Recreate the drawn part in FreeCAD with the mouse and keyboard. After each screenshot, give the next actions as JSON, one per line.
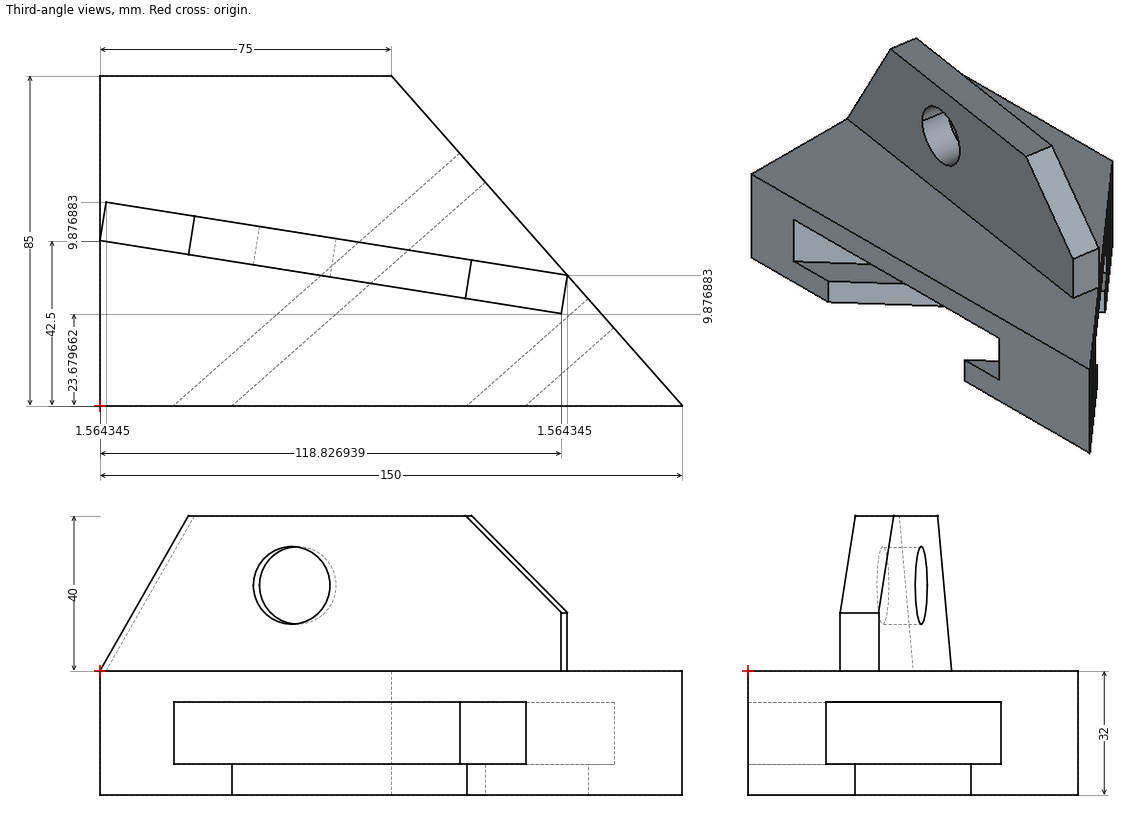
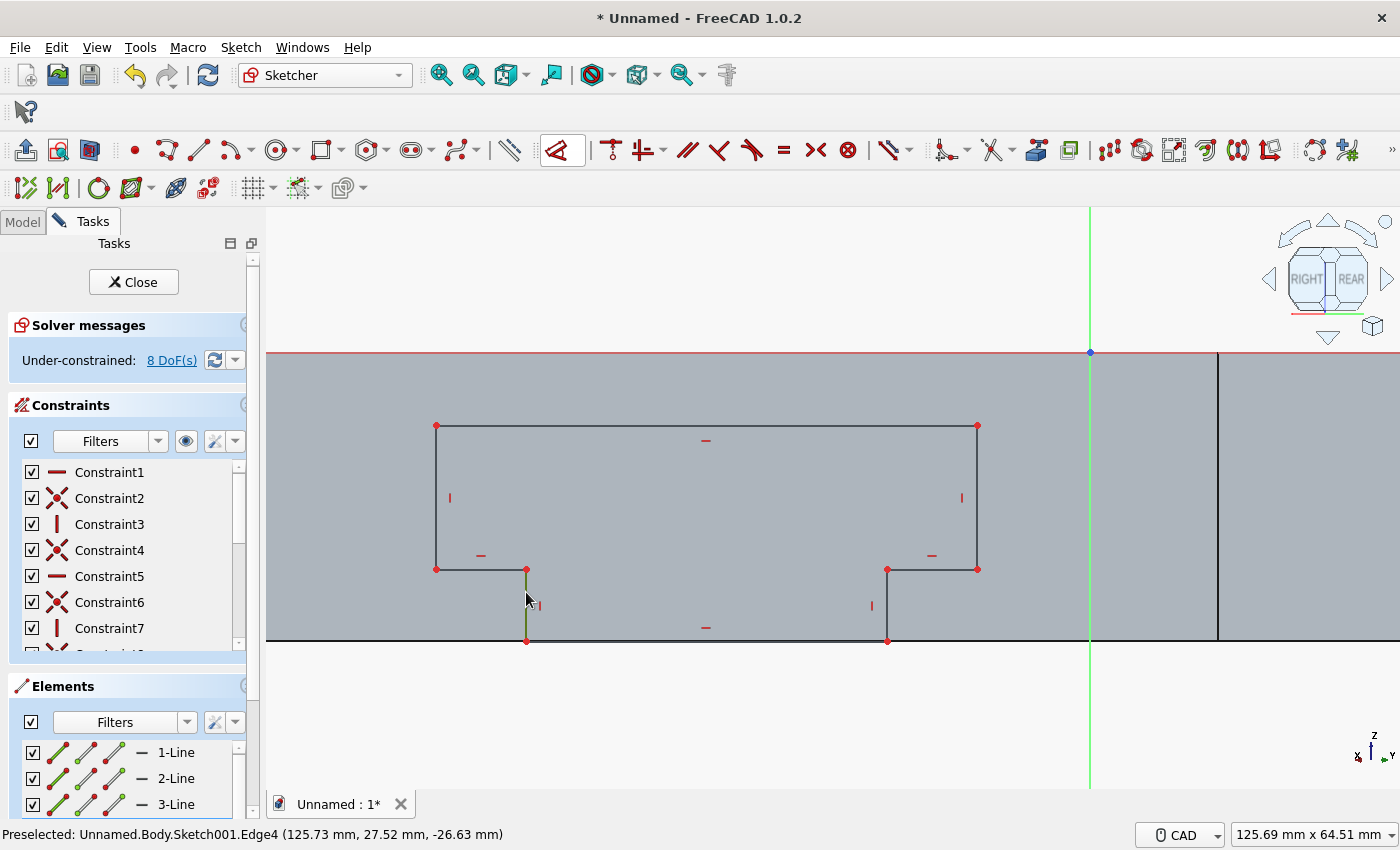
{"action": "key", "text": "i"}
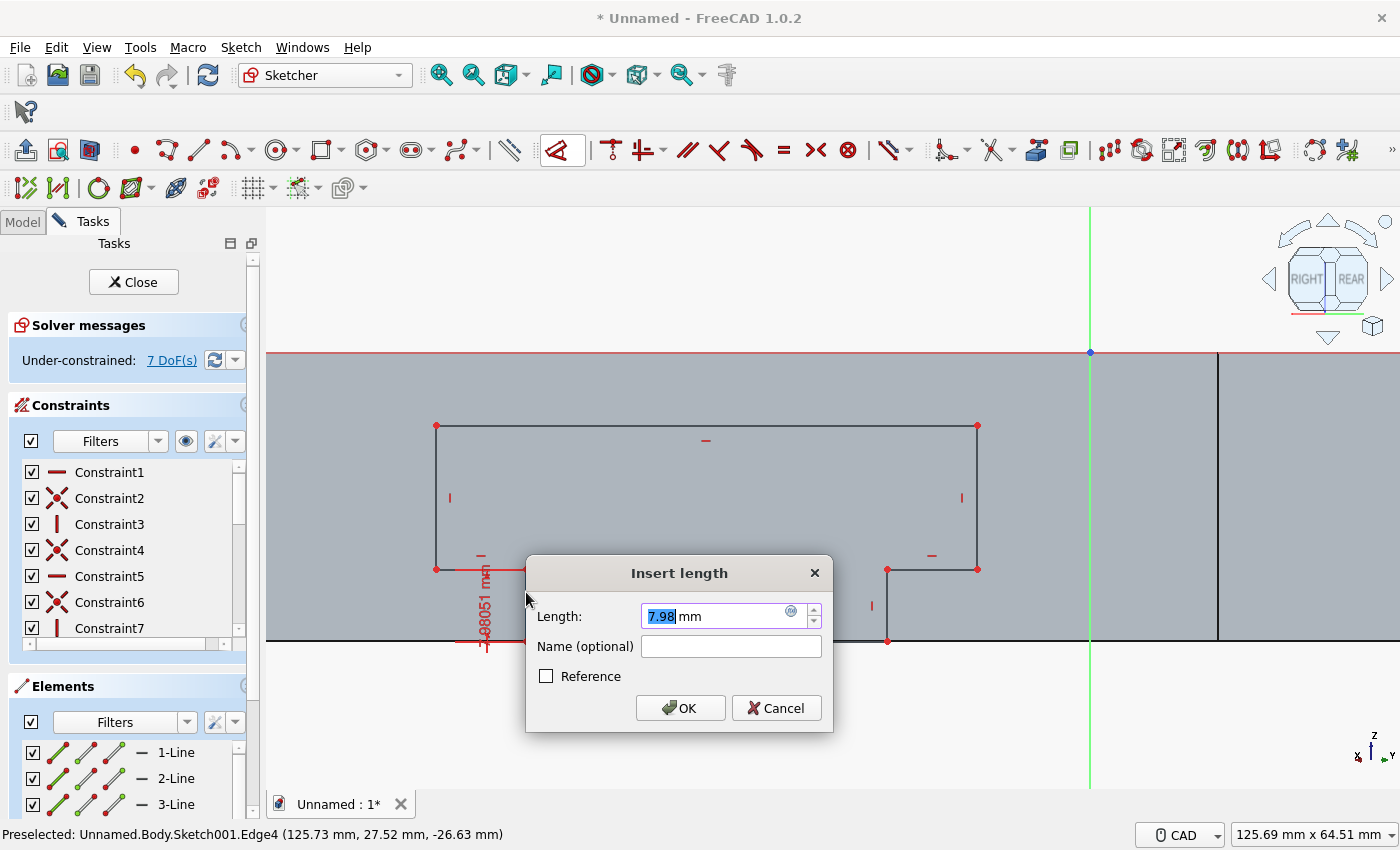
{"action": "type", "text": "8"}
{"action": "key", "text": "Return"}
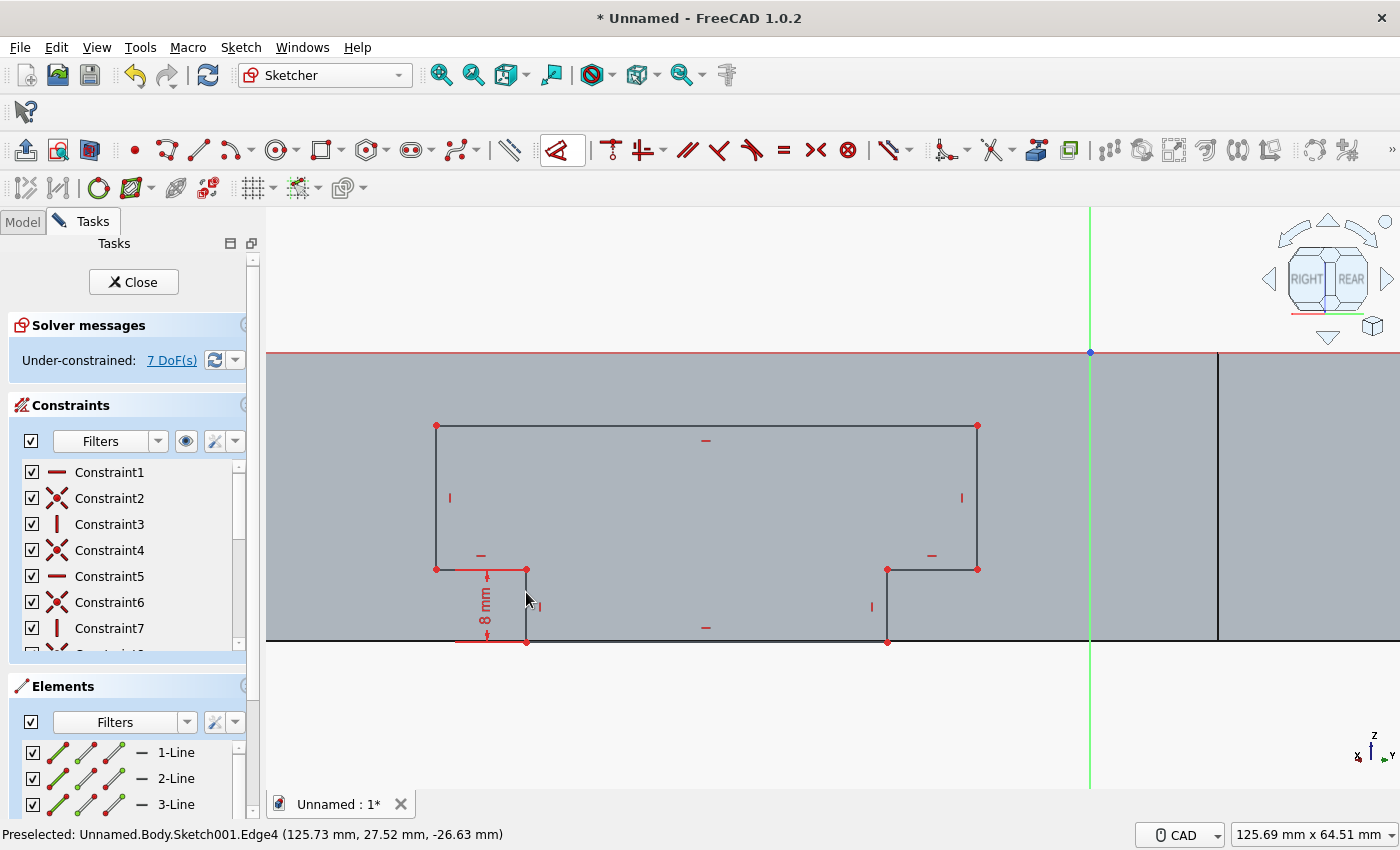
{"action": "left_click", "coordinate": [887, 621]}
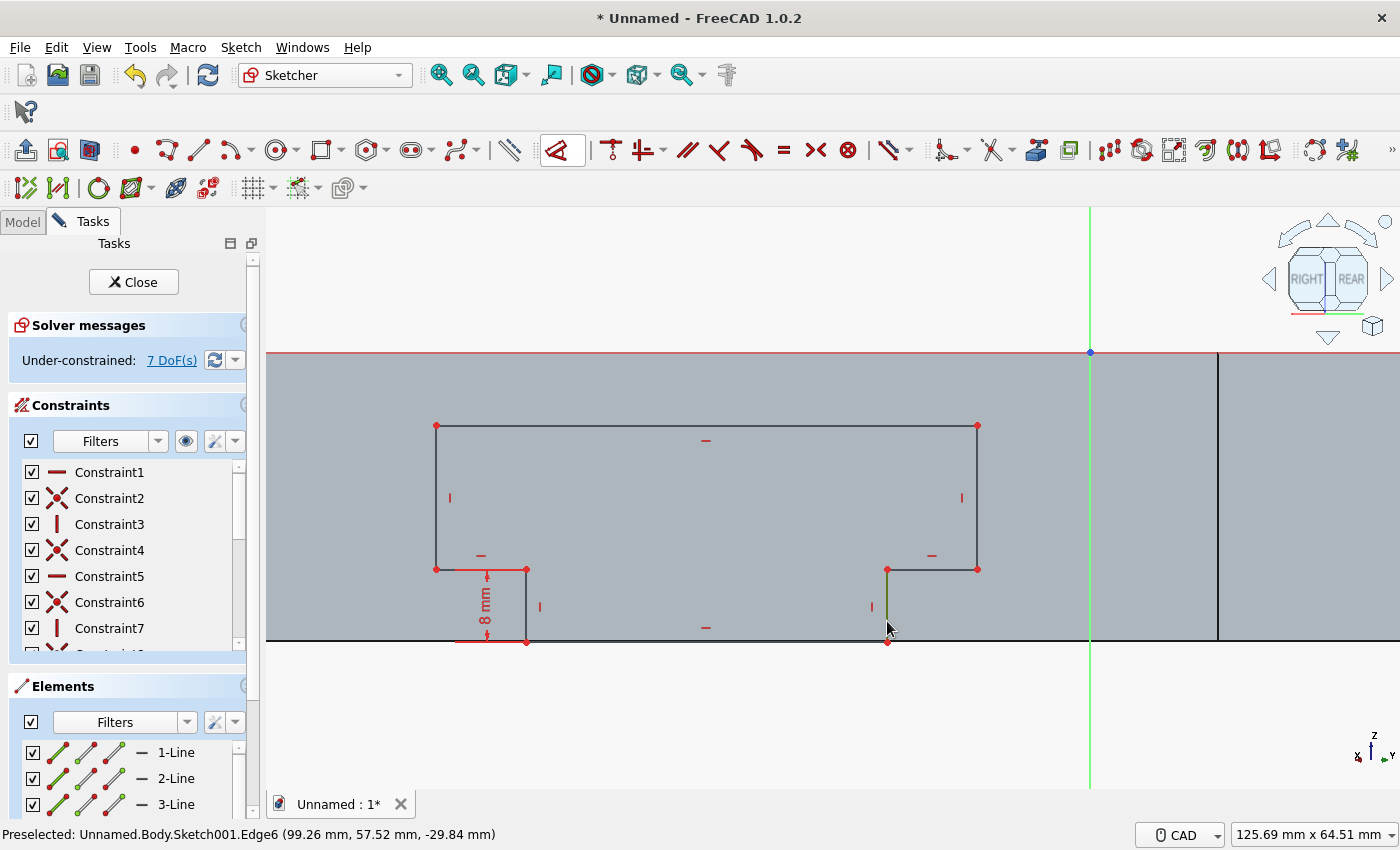
{"action": "key", "text": "i"}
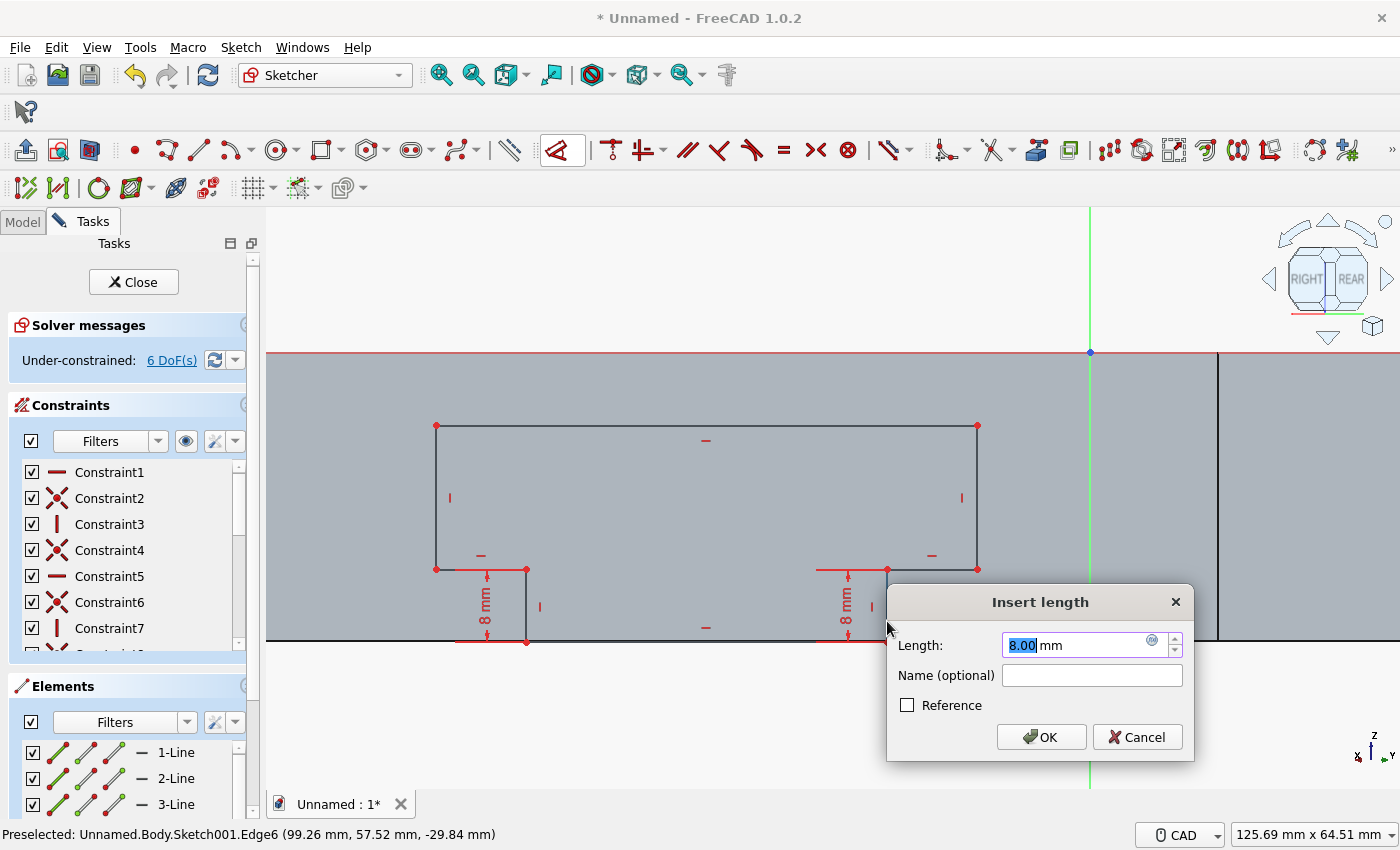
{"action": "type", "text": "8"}
{"action": "key", "text": "Return"}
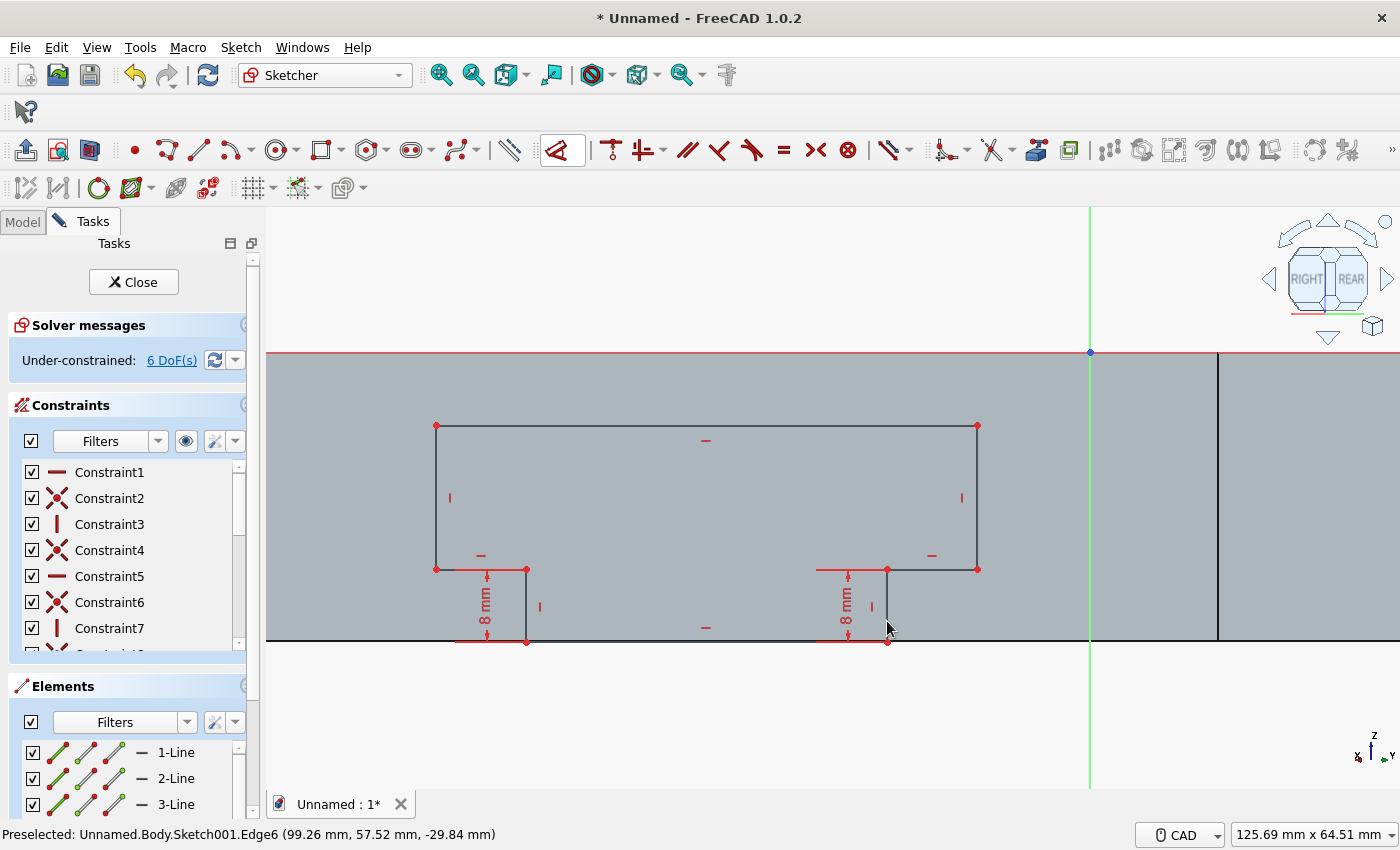
{"action": "left_click", "coordinate": [815, 426]}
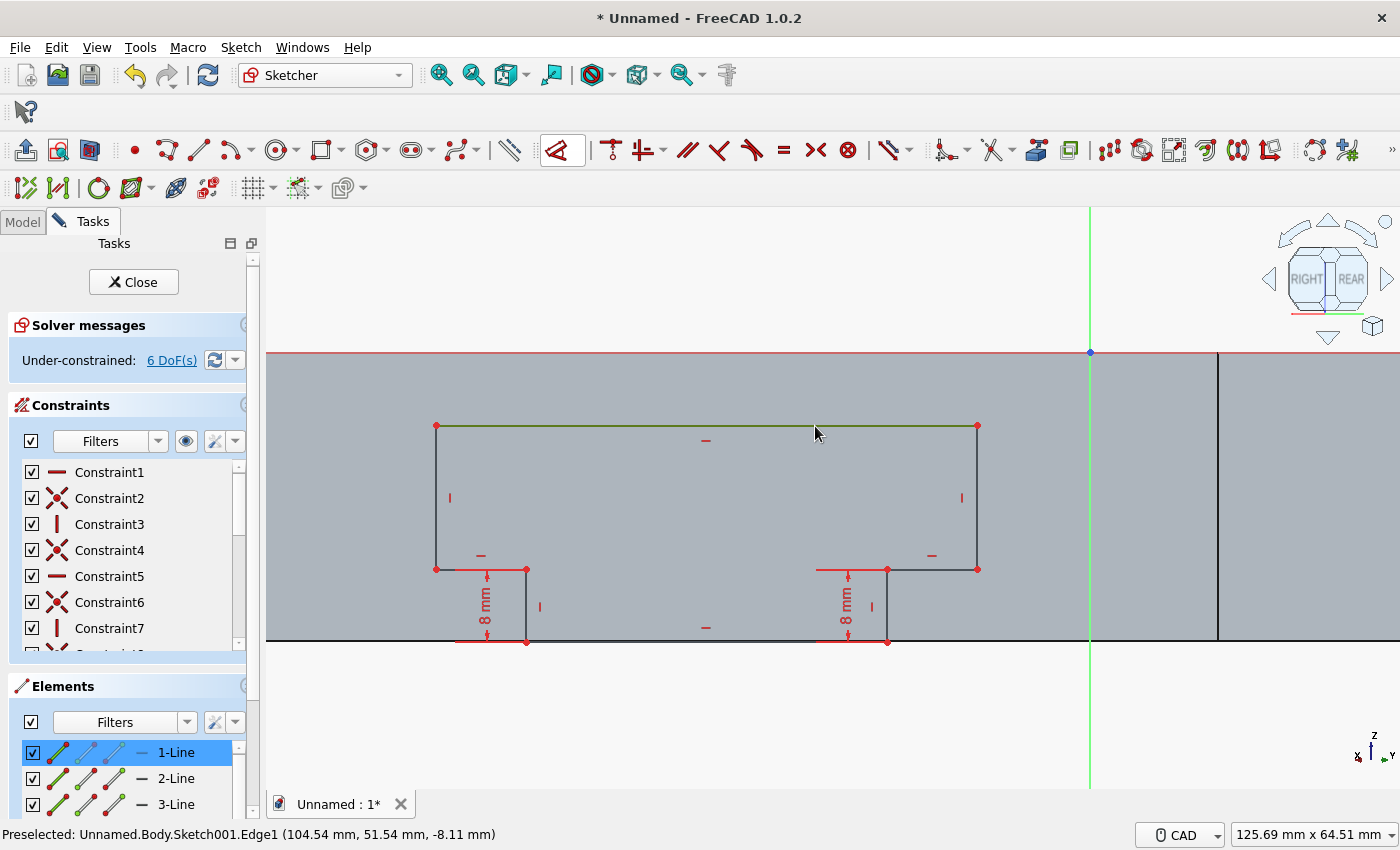
{"action": "key", "text": "l"}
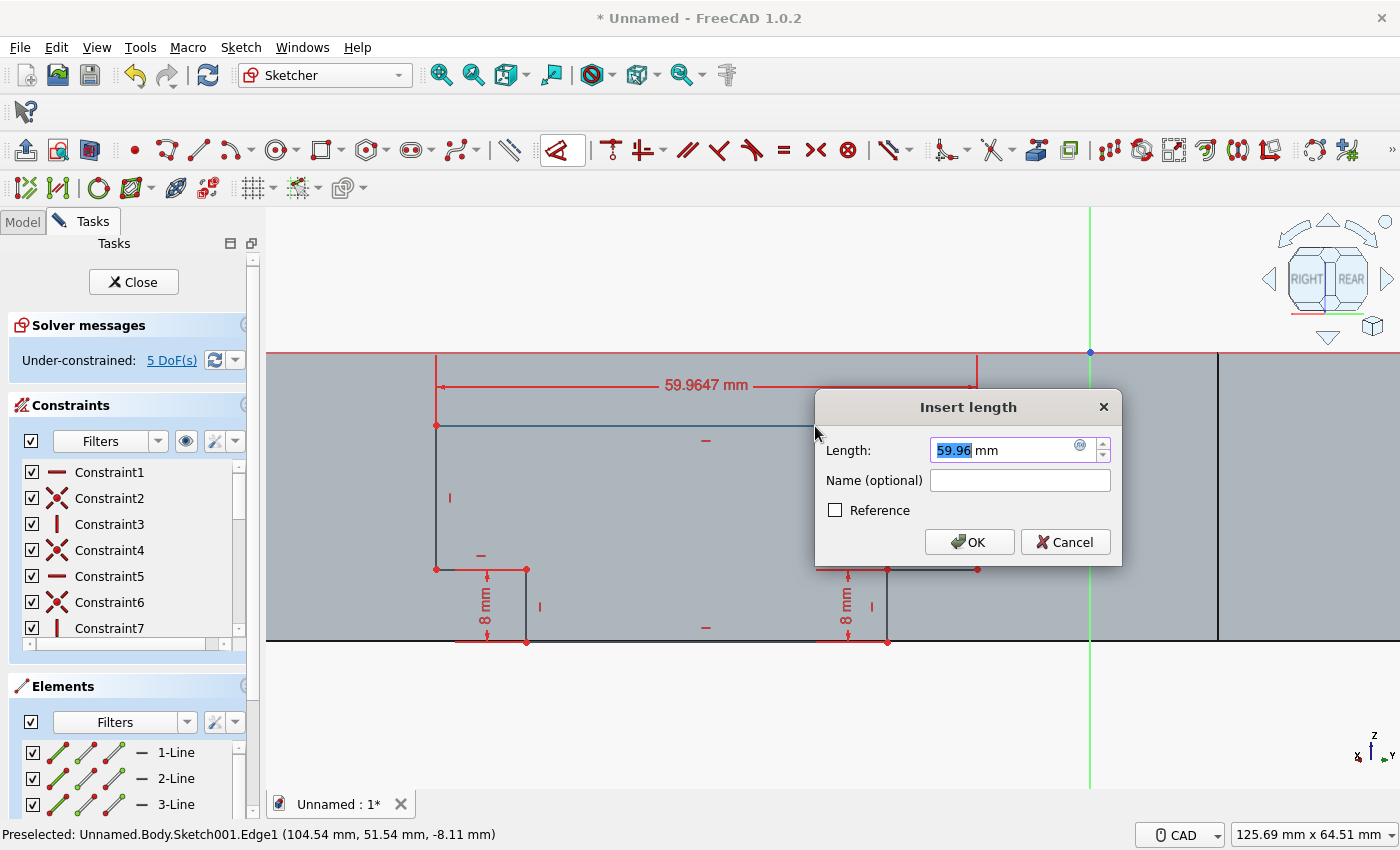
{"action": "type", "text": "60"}
{"action": "key", "text": "Return"}